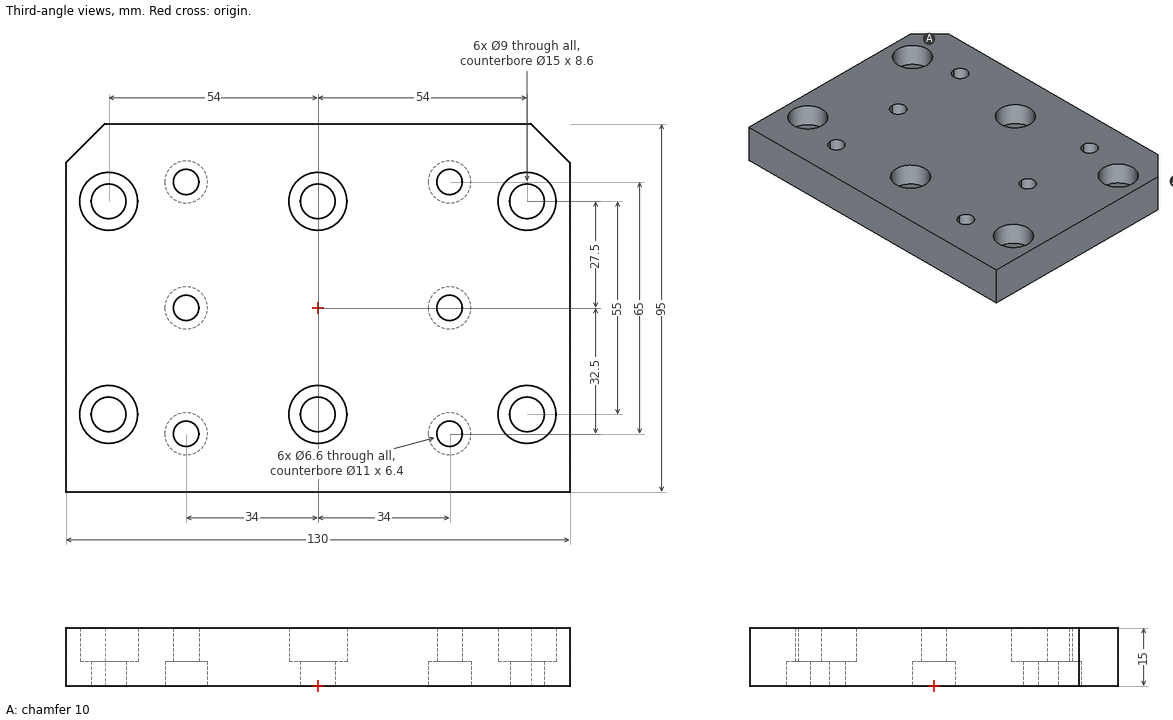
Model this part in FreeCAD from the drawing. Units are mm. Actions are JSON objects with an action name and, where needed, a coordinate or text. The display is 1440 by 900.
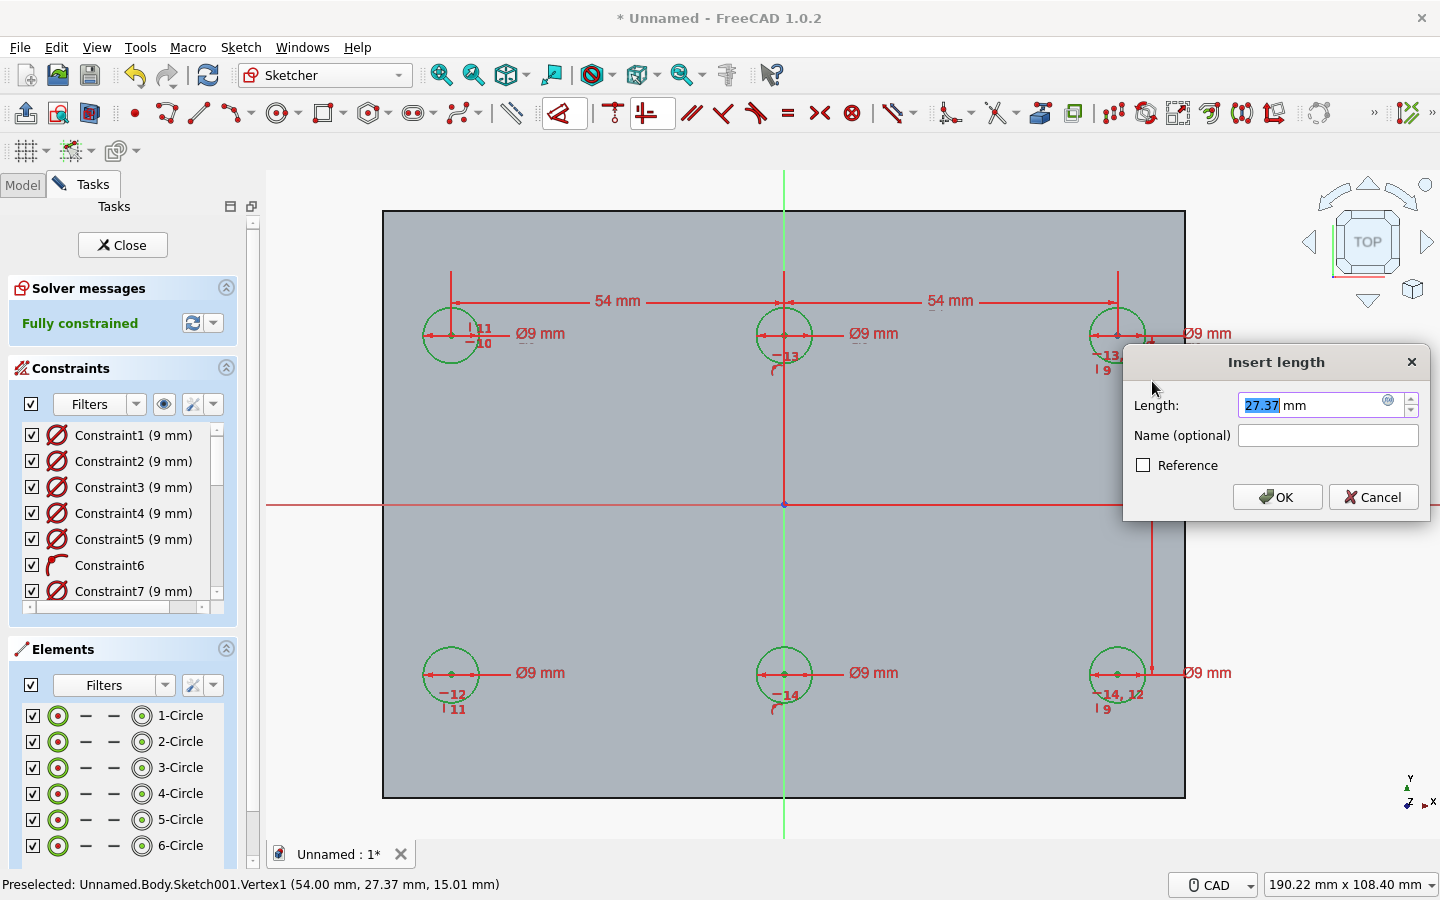
{"action": "type", "text": "27.5"}
{"action": "key", "text": "Return"}
{"action": "key", "text": "Escape"}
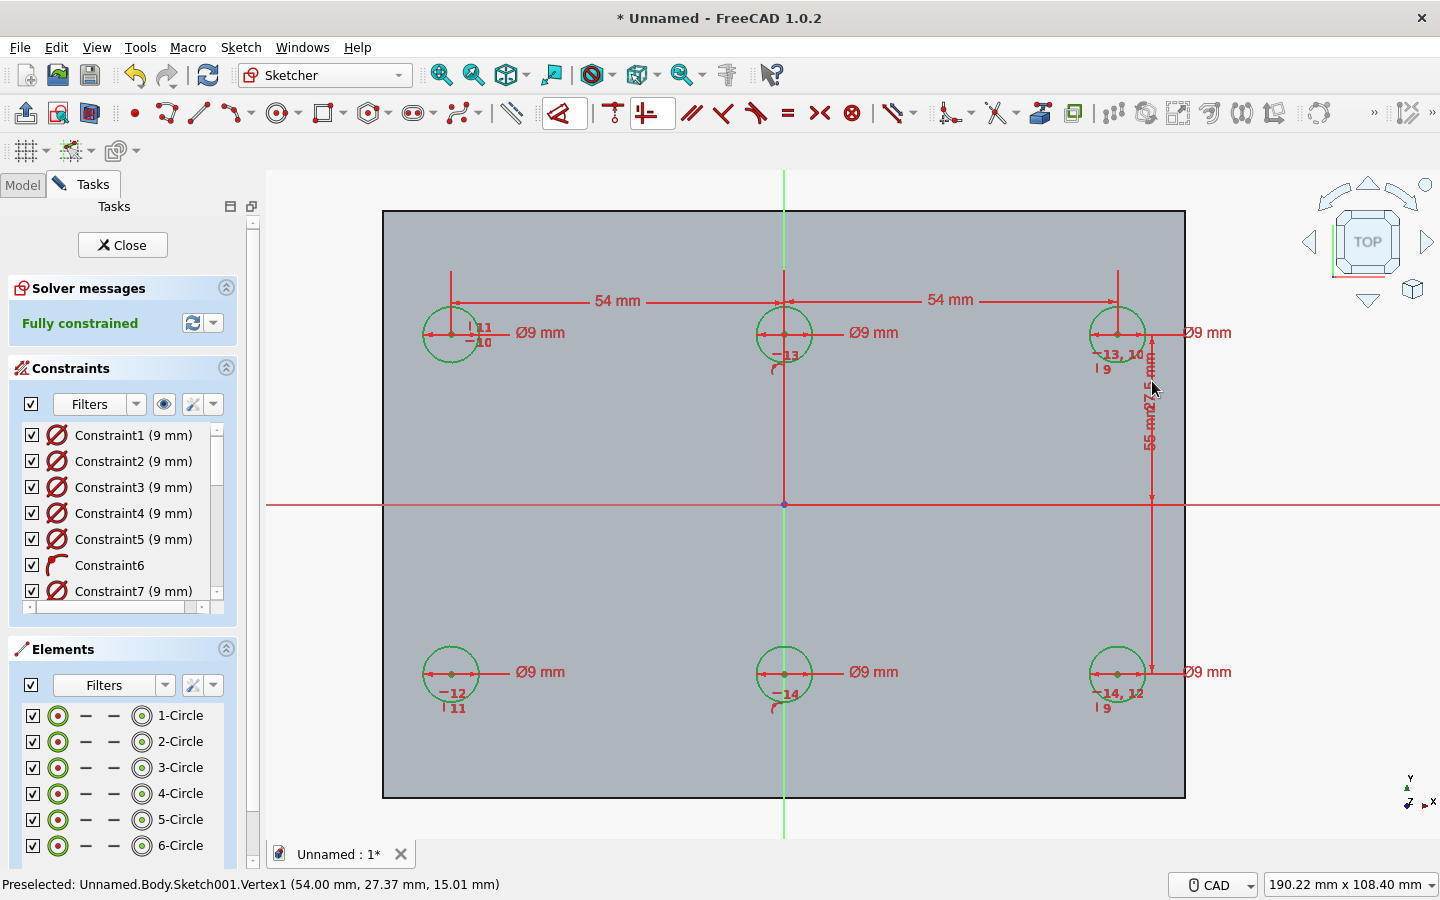
{"action": "left_click", "coordinate": [123, 245]}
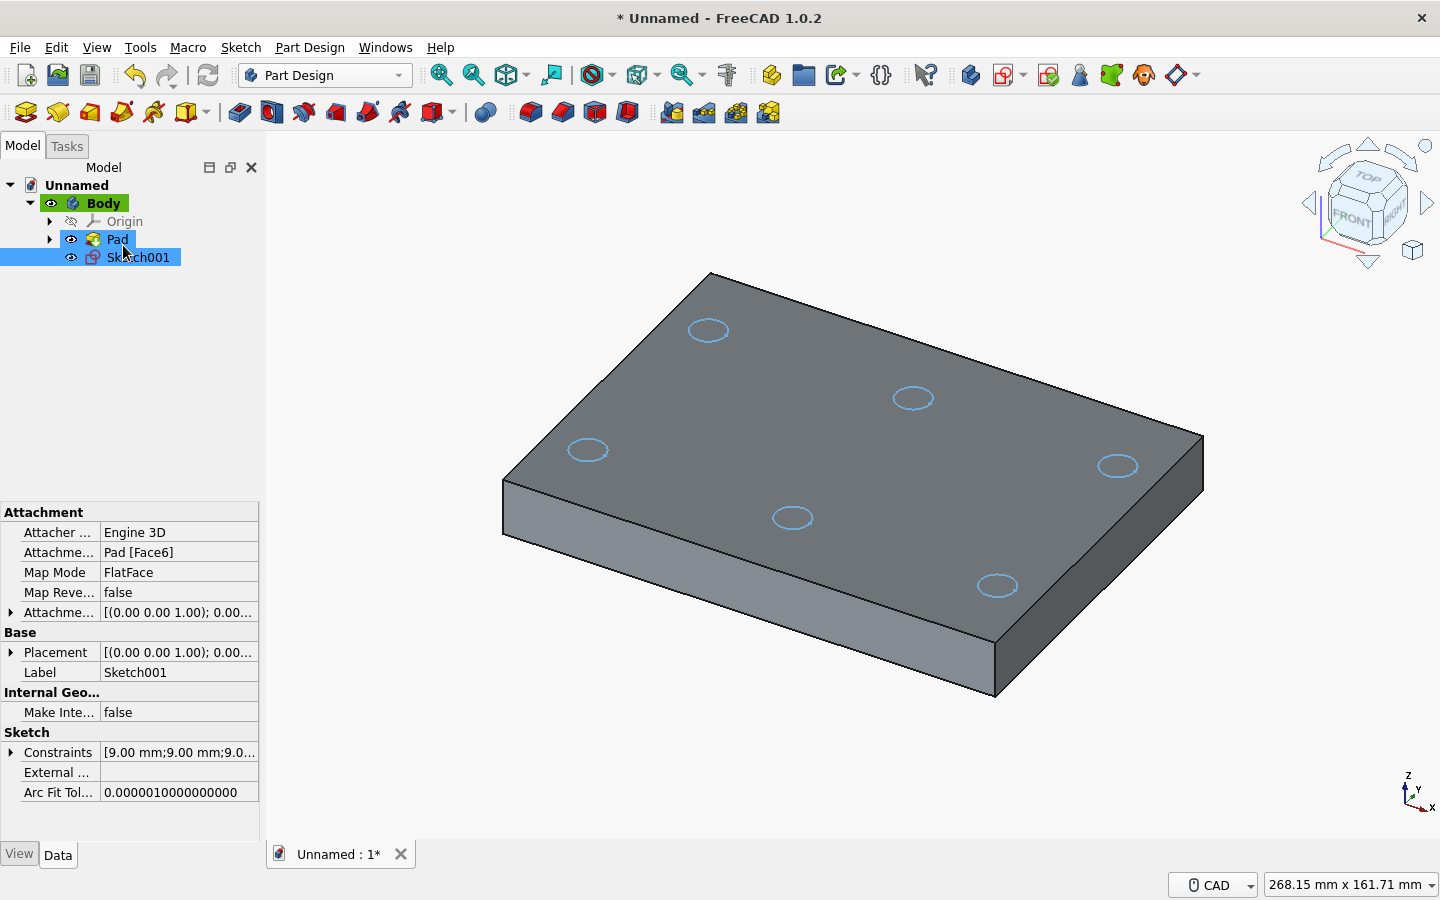
{"action": "left_click", "coordinate": [272, 112]}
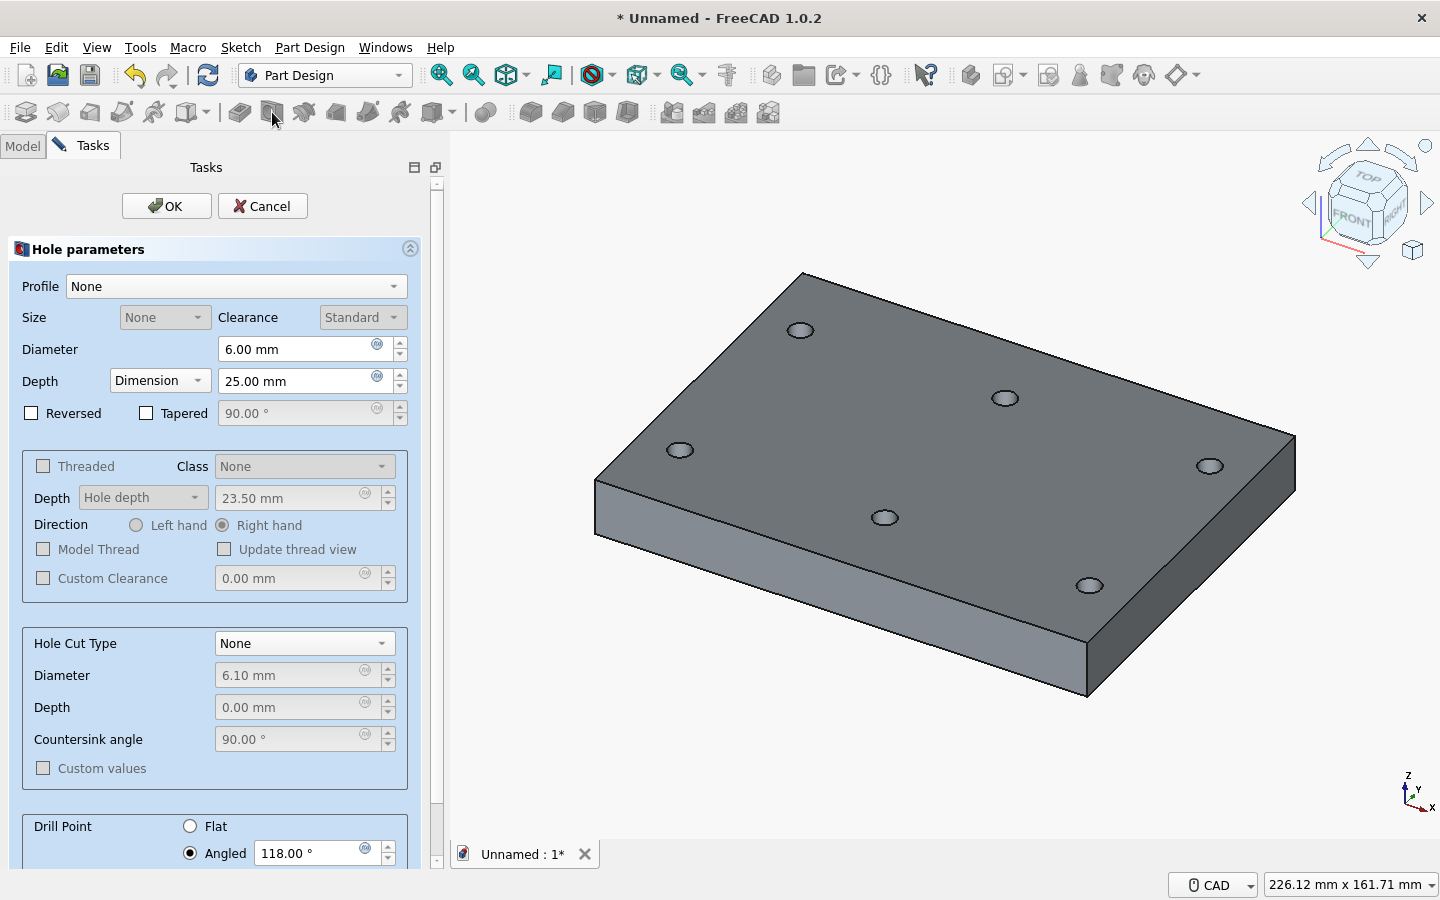
{"action": "triple_click", "coordinate": [305, 349]}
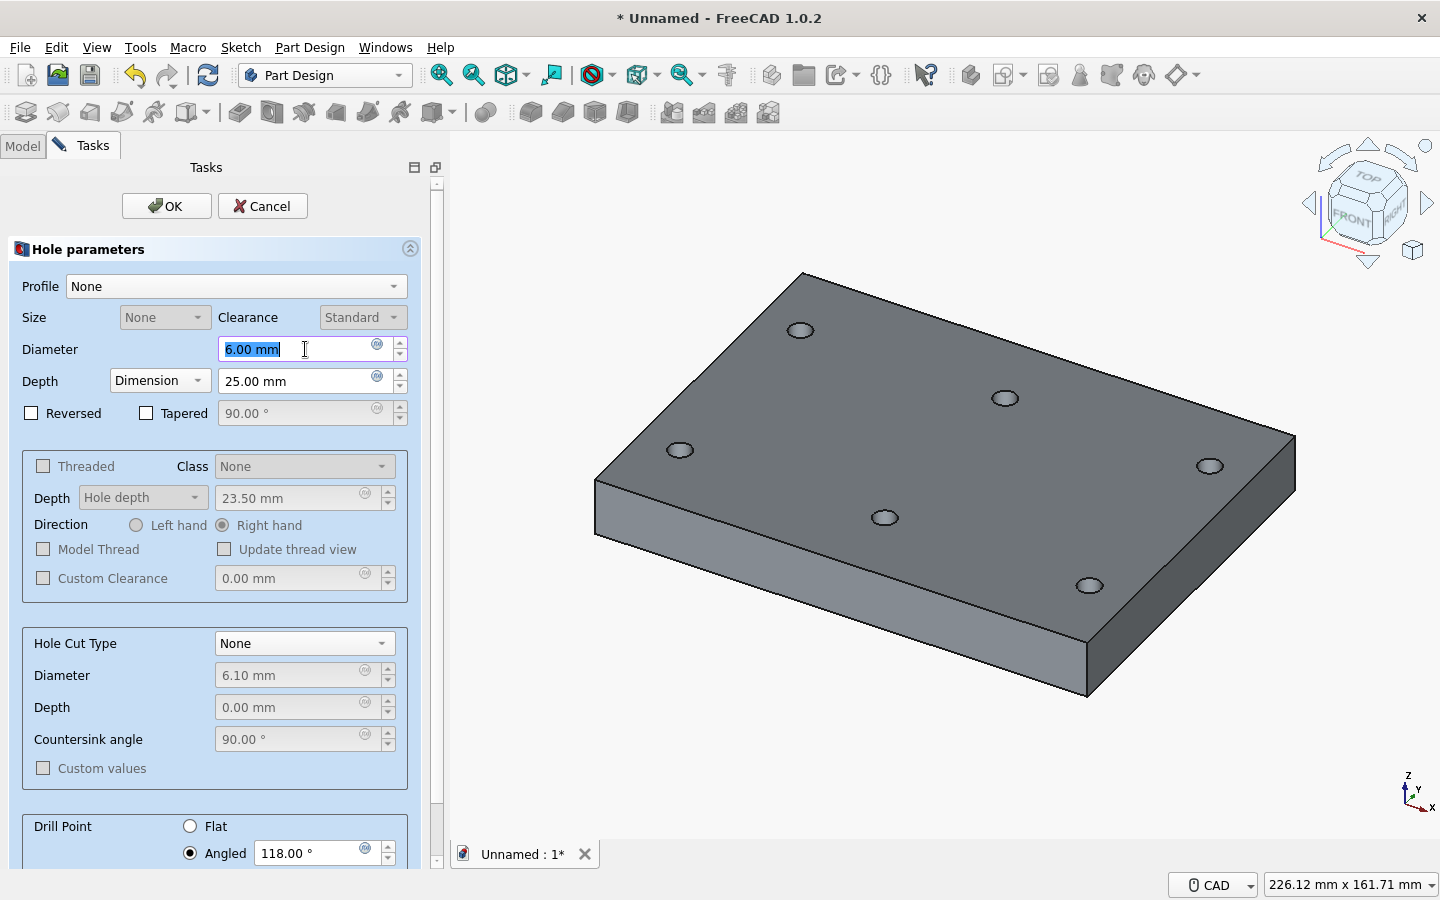
{"action": "type", "text": "9"}
{"action": "key", "text": "Tab"}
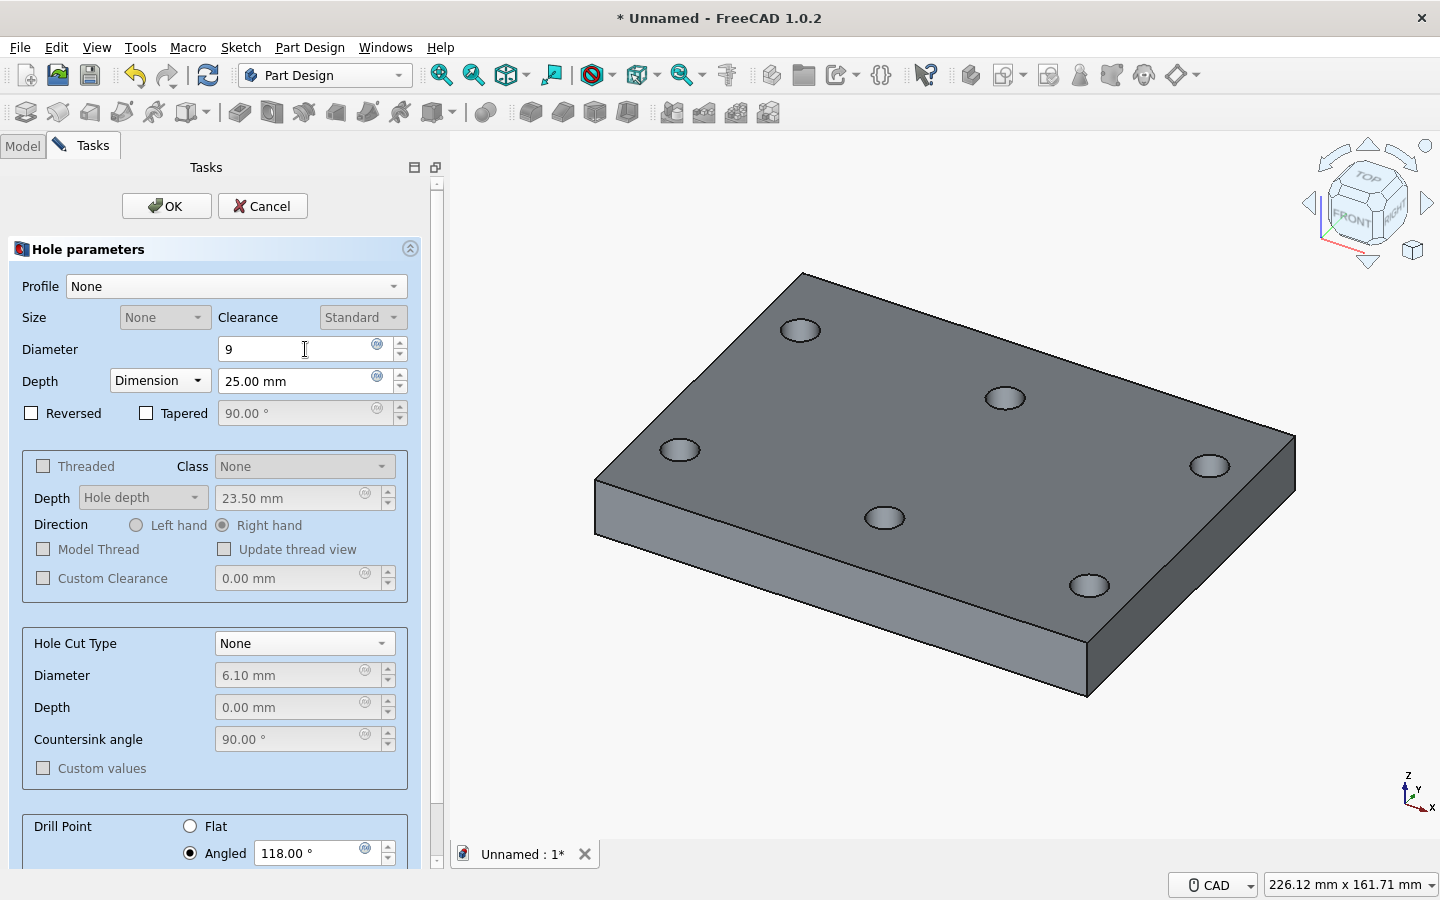
{"action": "left_click", "coordinate": [161, 380]}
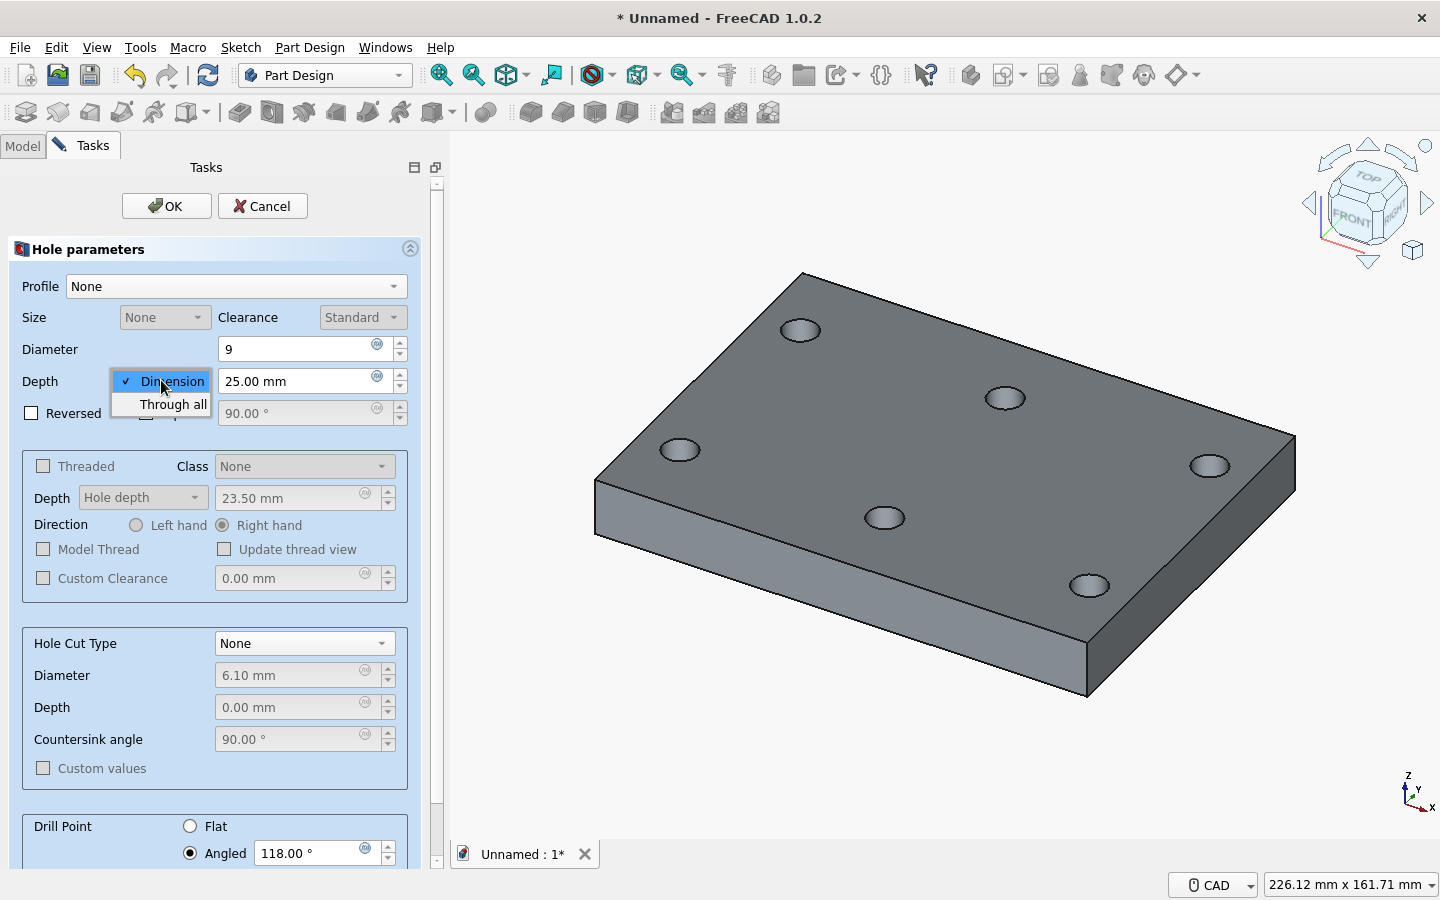
{"action": "left_click", "coordinate": [160, 404]}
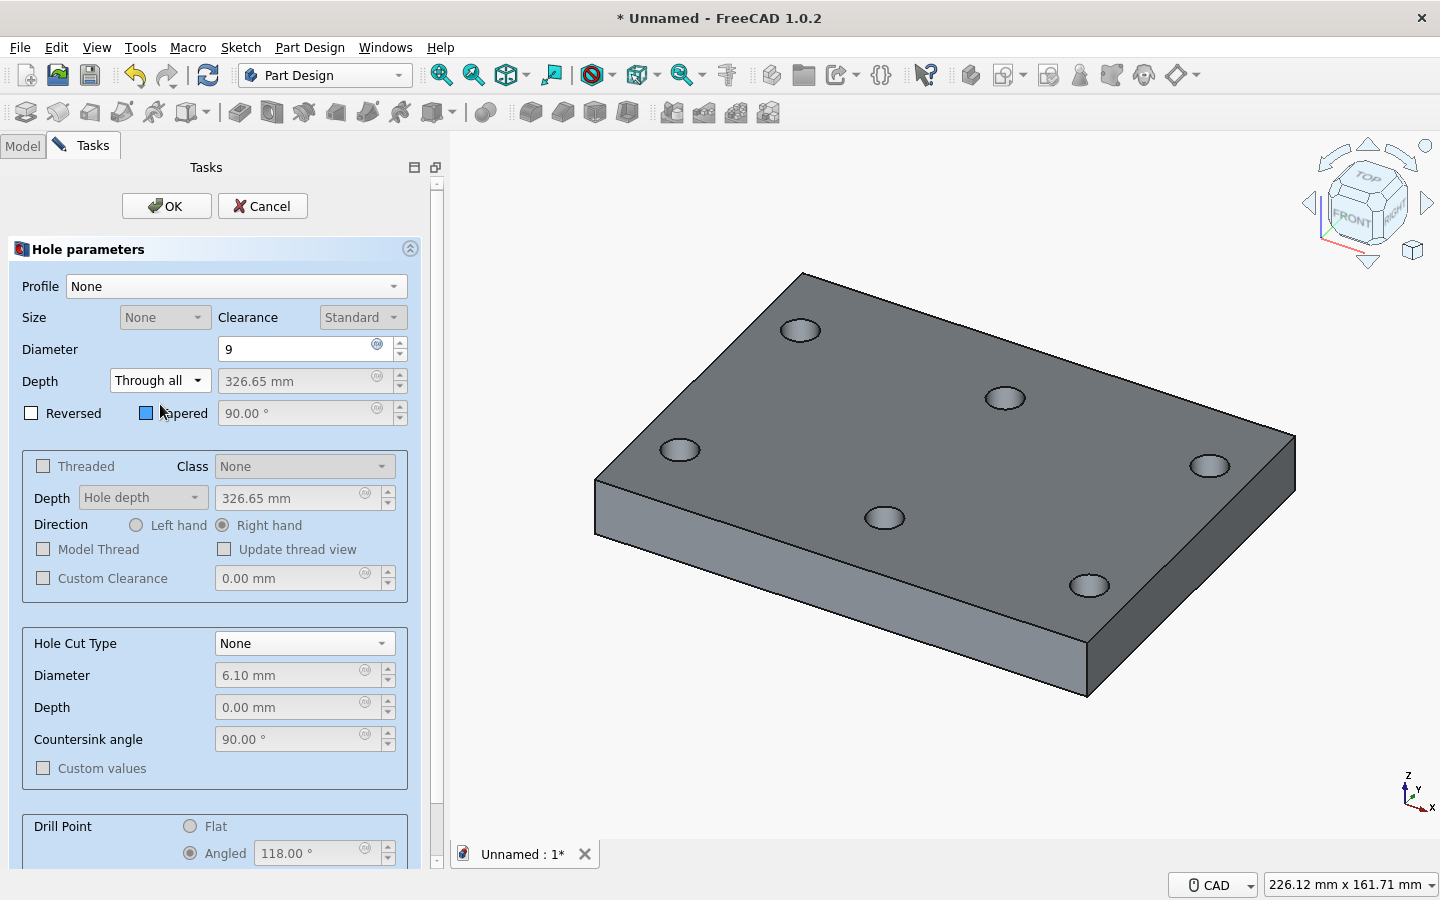
{"action": "left_click", "coordinate": [306, 644]}